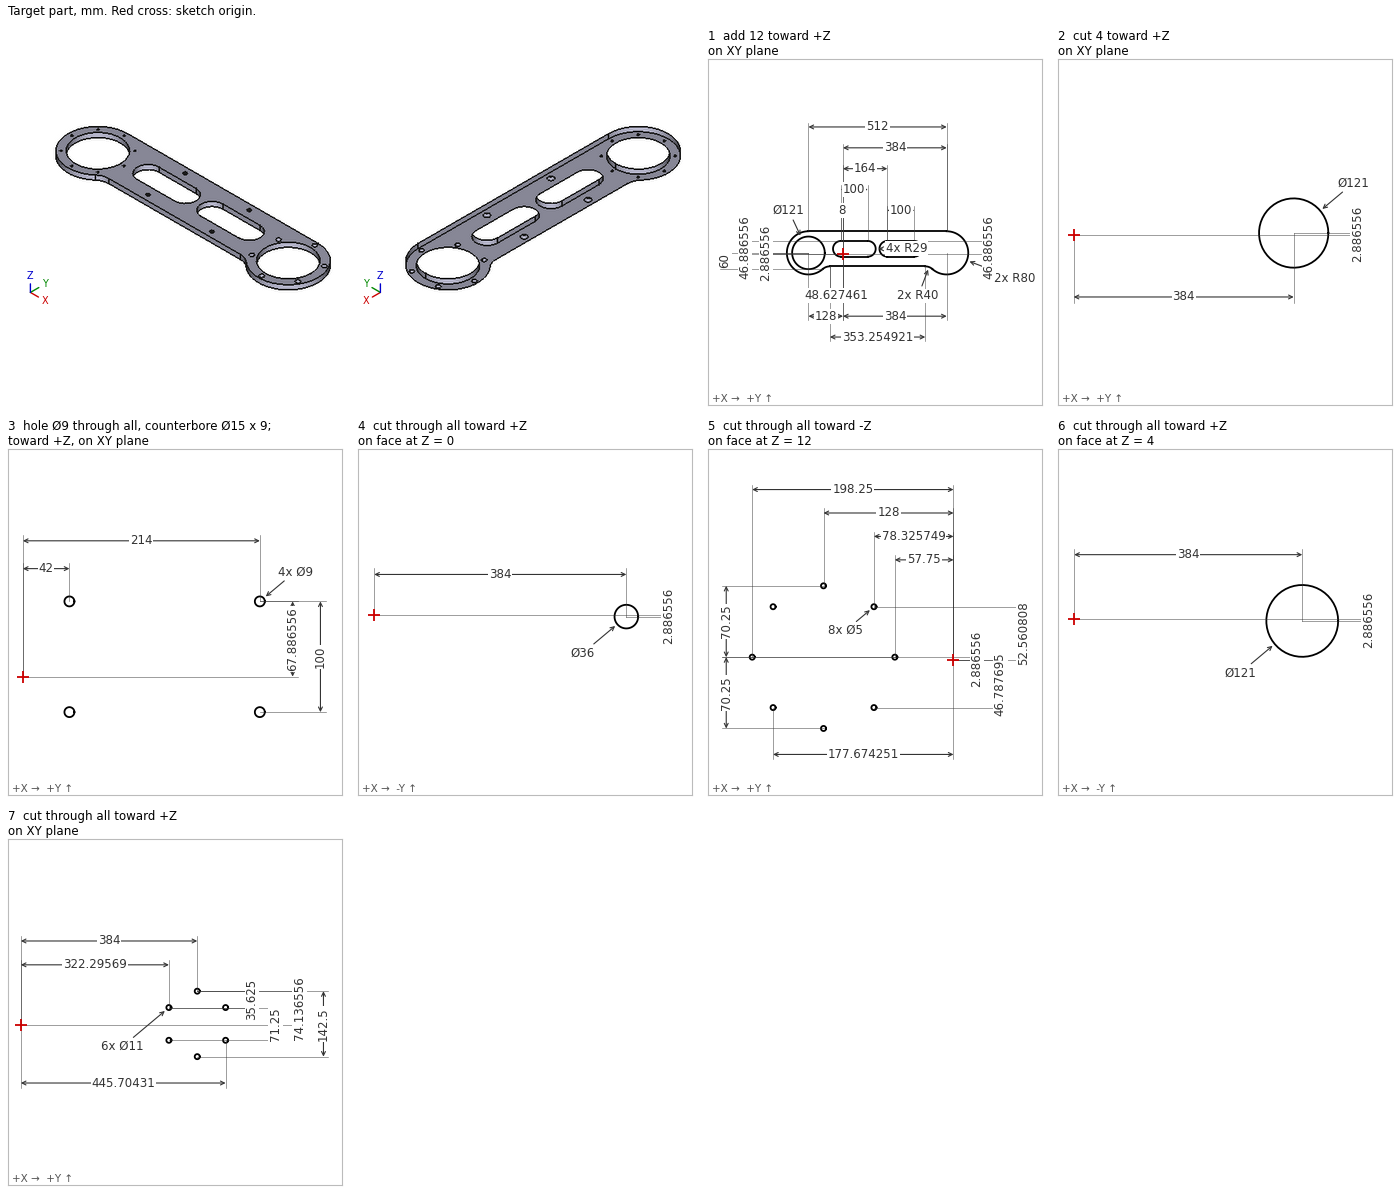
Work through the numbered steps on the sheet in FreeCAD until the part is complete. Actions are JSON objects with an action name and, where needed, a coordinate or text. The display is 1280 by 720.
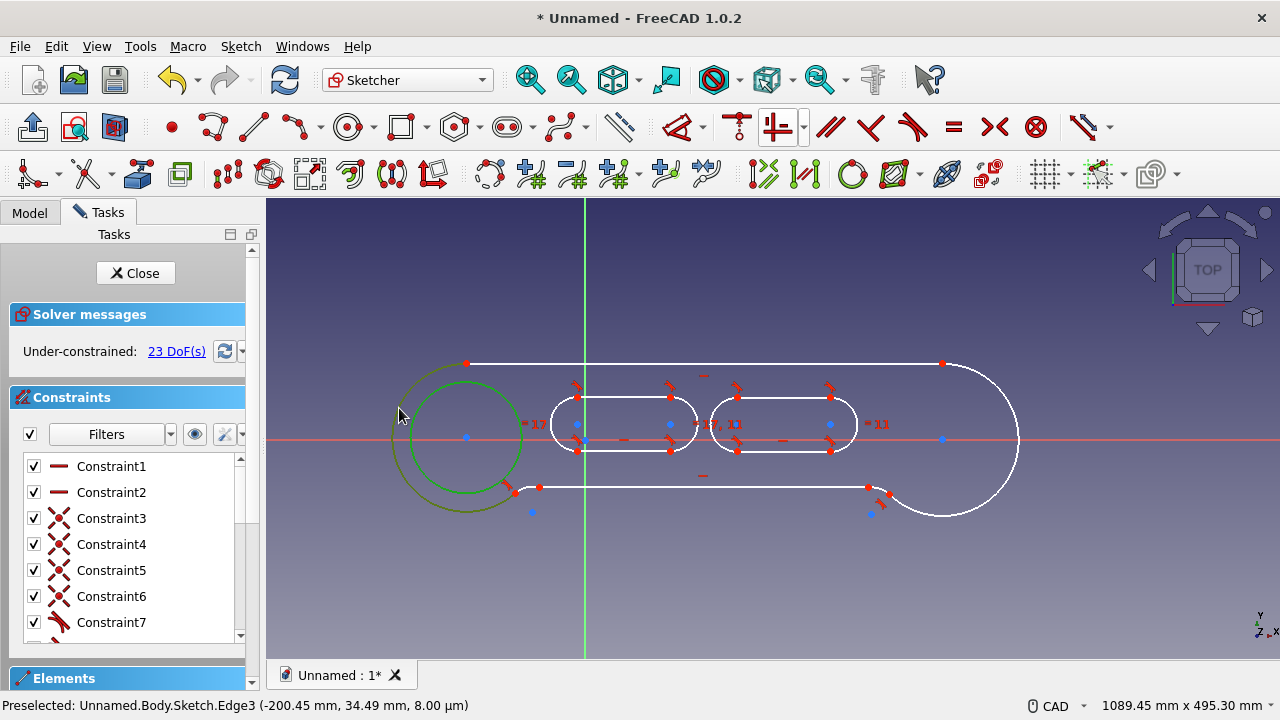
{"action": "left_click", "coordinate": [737, 128]}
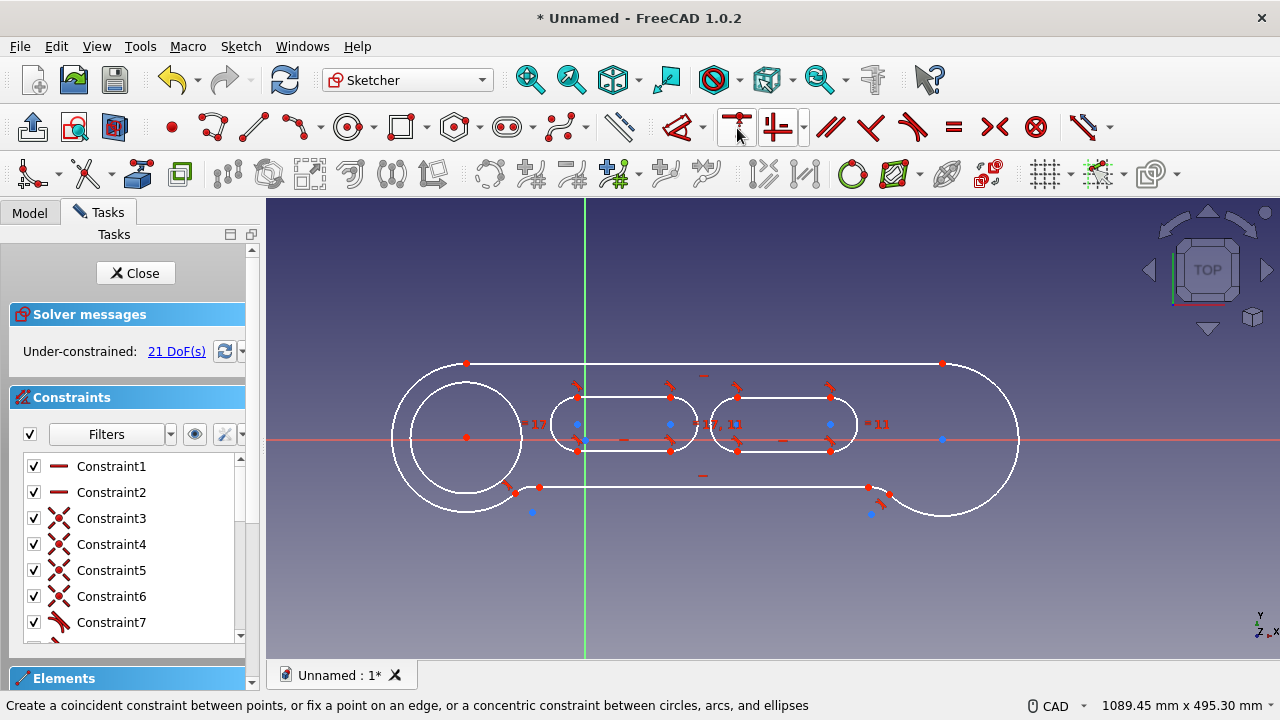
{"action": "left_click", "coordinate": [527, 487]}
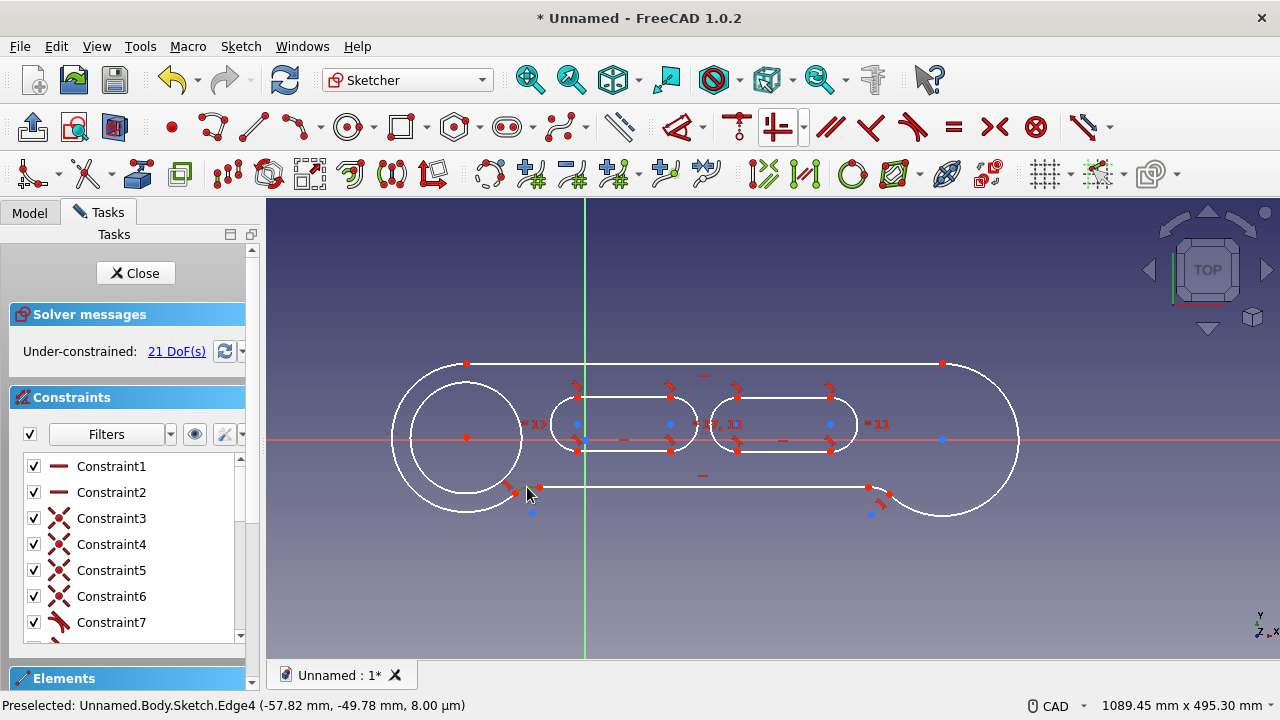
{"action": "left_click", "coordinate": [880, 489]}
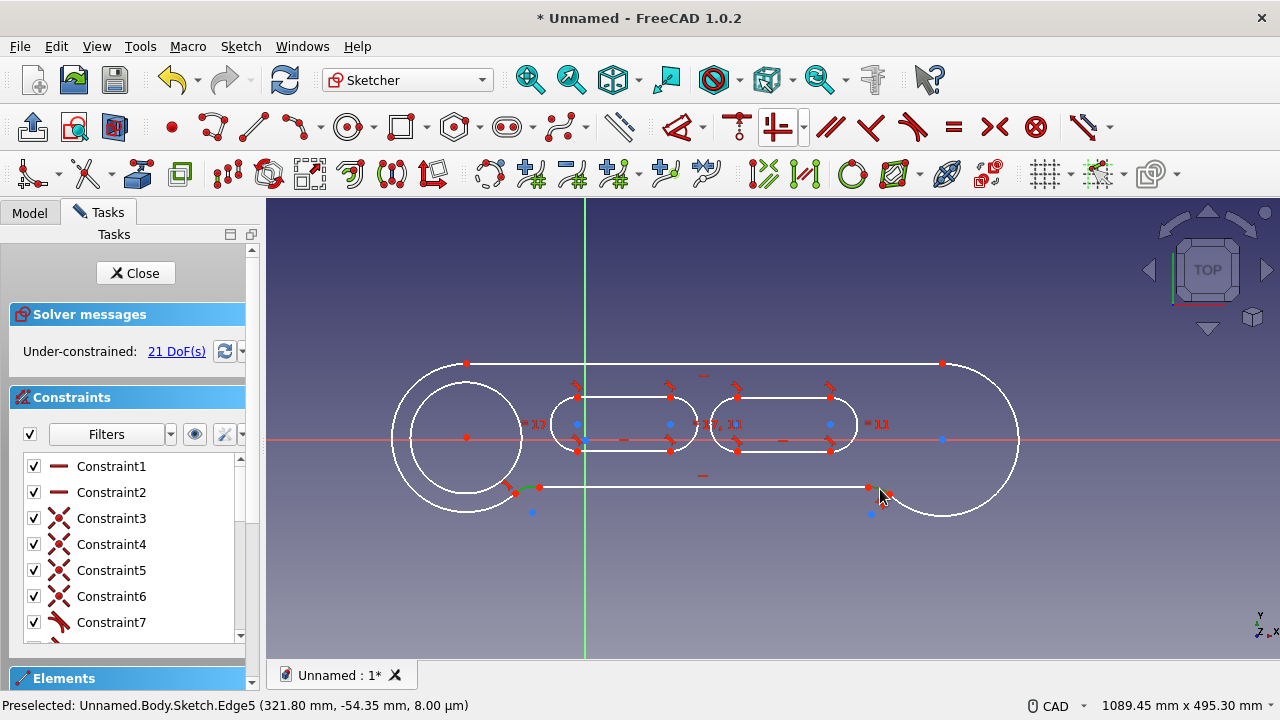
{"action": "left_click", "coordinate": [954, 128]}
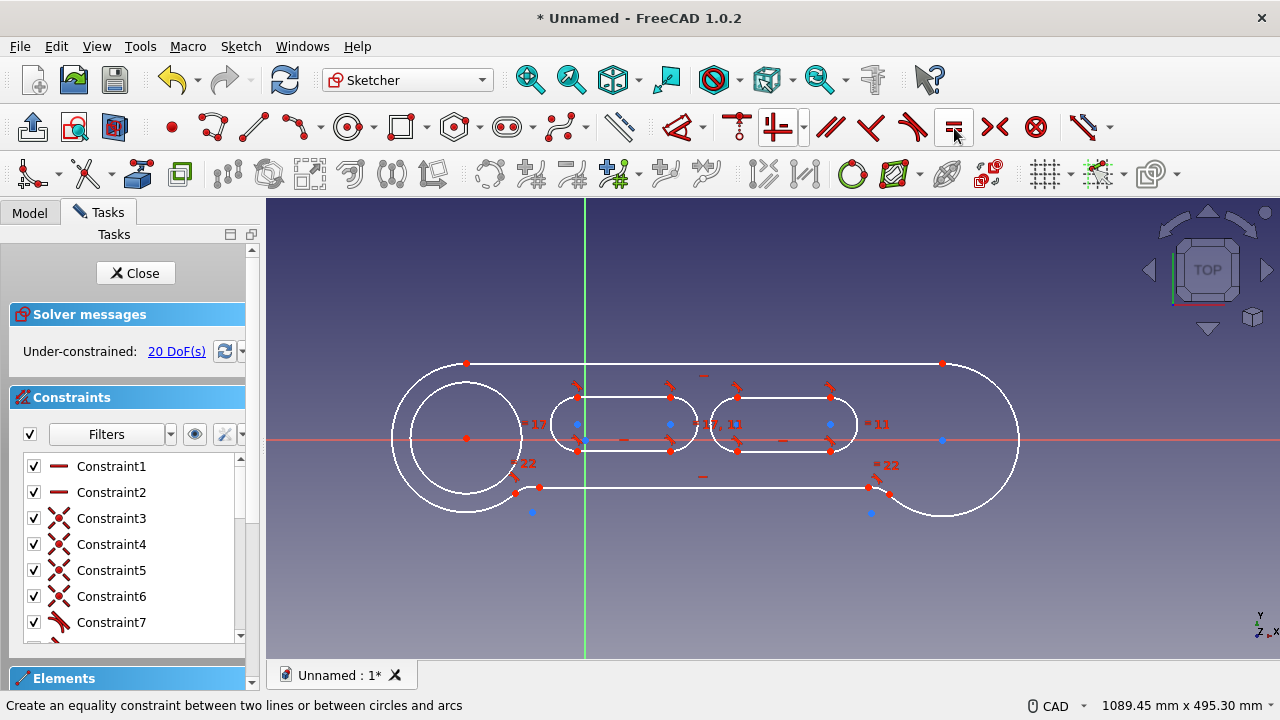
{"action": "left_click", "coordinate": [398, 408]}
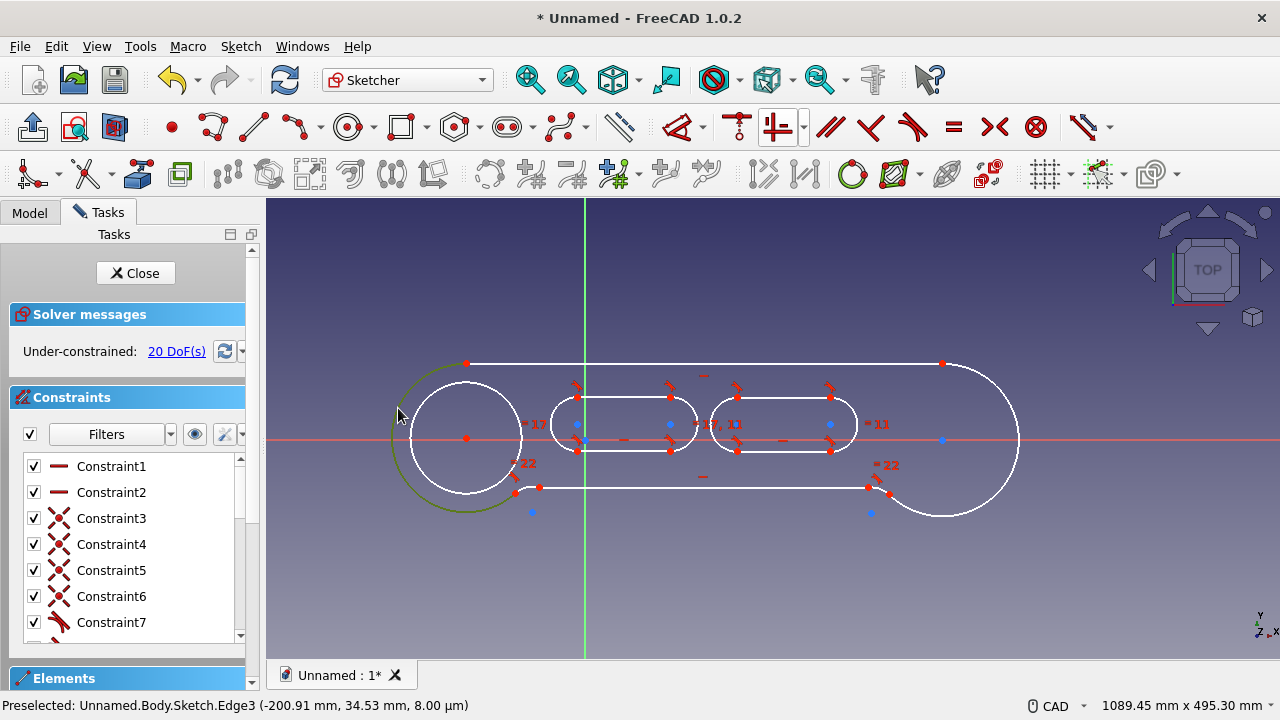
{"action": "left_click", "coordinate": [972, 510]}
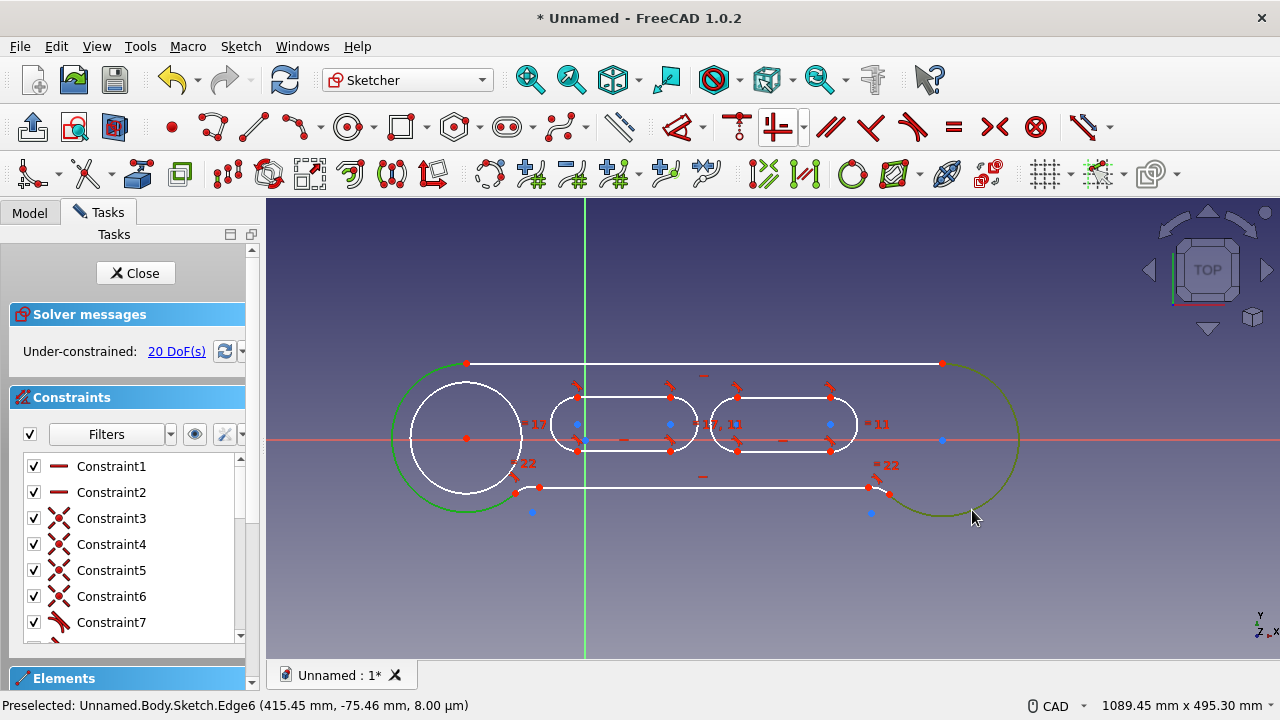
{"action": "left_click", "coordinate": [954, 128]}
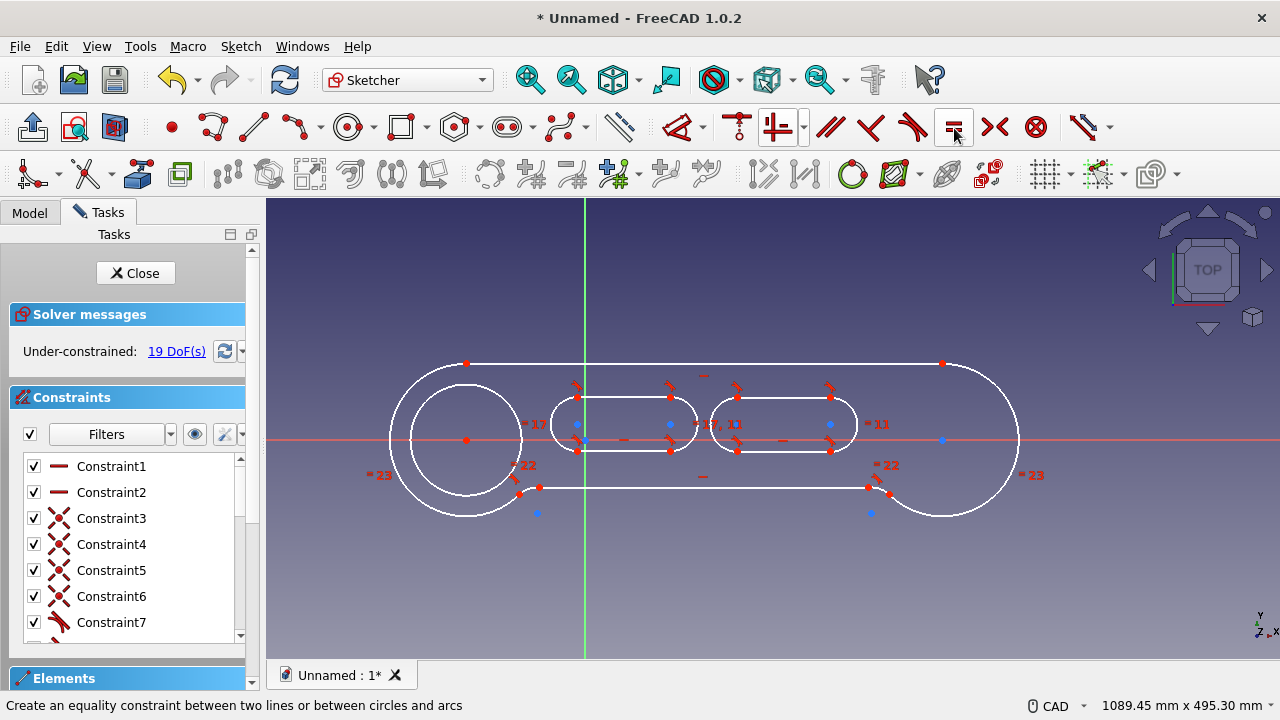
{"action": "left_click", "coordinate": [716, 409]}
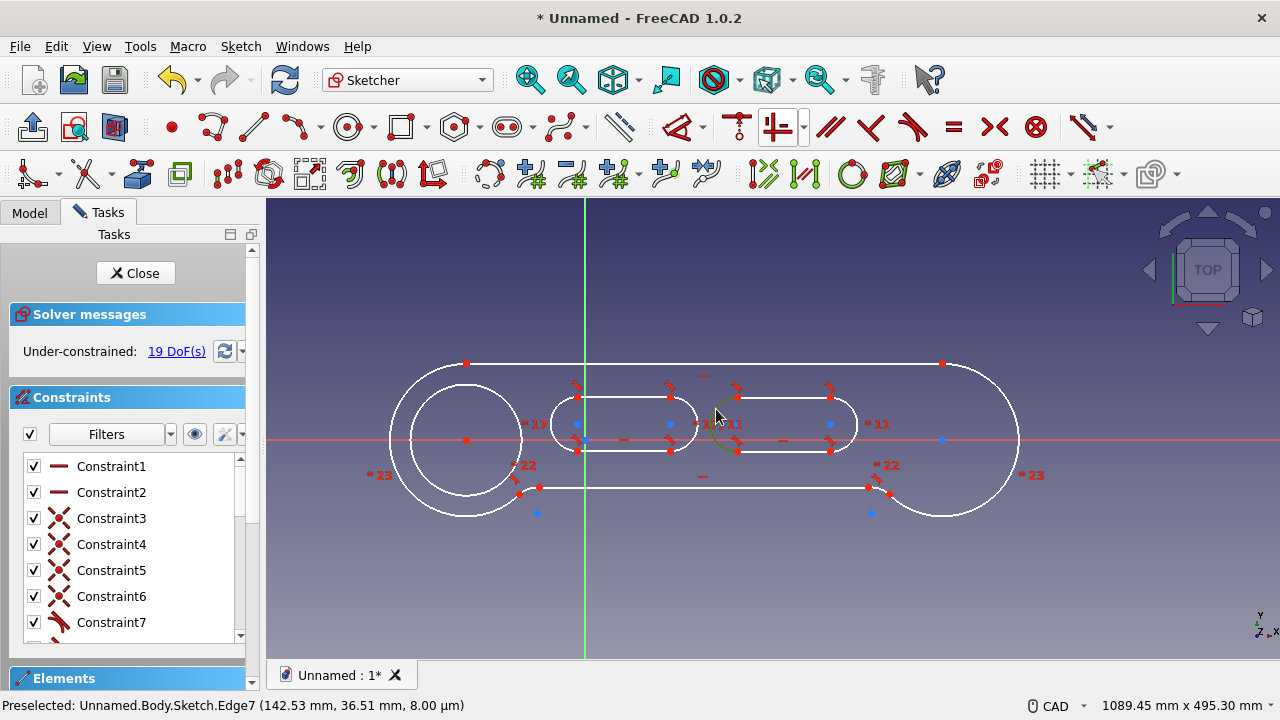
{"action": "left_click", "coordinate": [556, 408]}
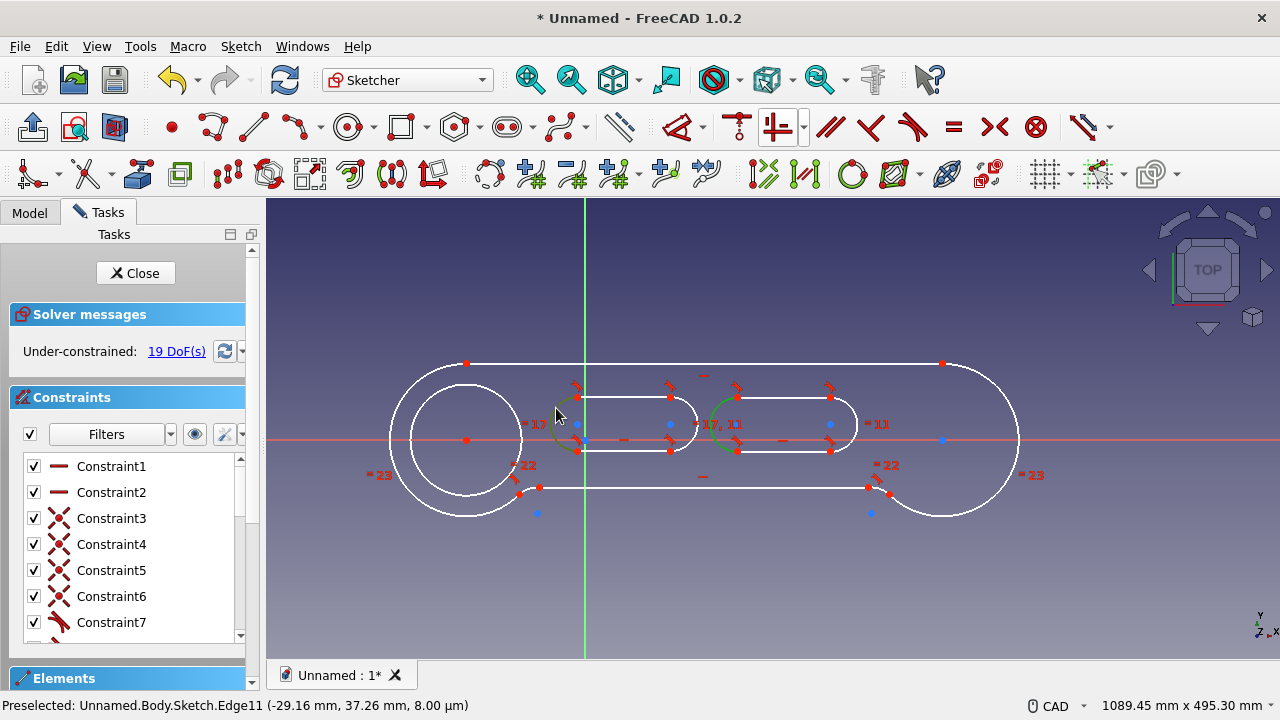
{"action": "left_click", "coordinate": [954, 128]}